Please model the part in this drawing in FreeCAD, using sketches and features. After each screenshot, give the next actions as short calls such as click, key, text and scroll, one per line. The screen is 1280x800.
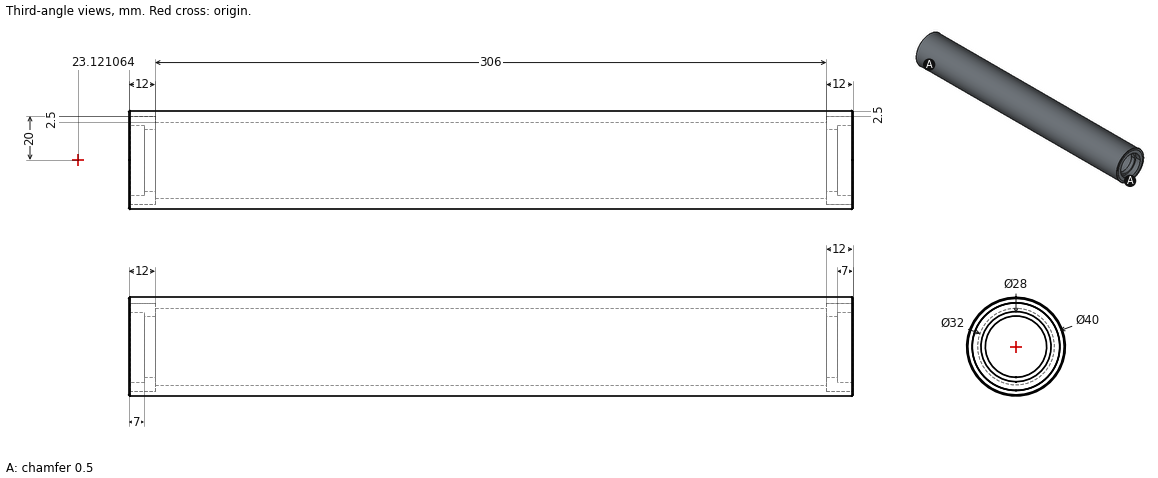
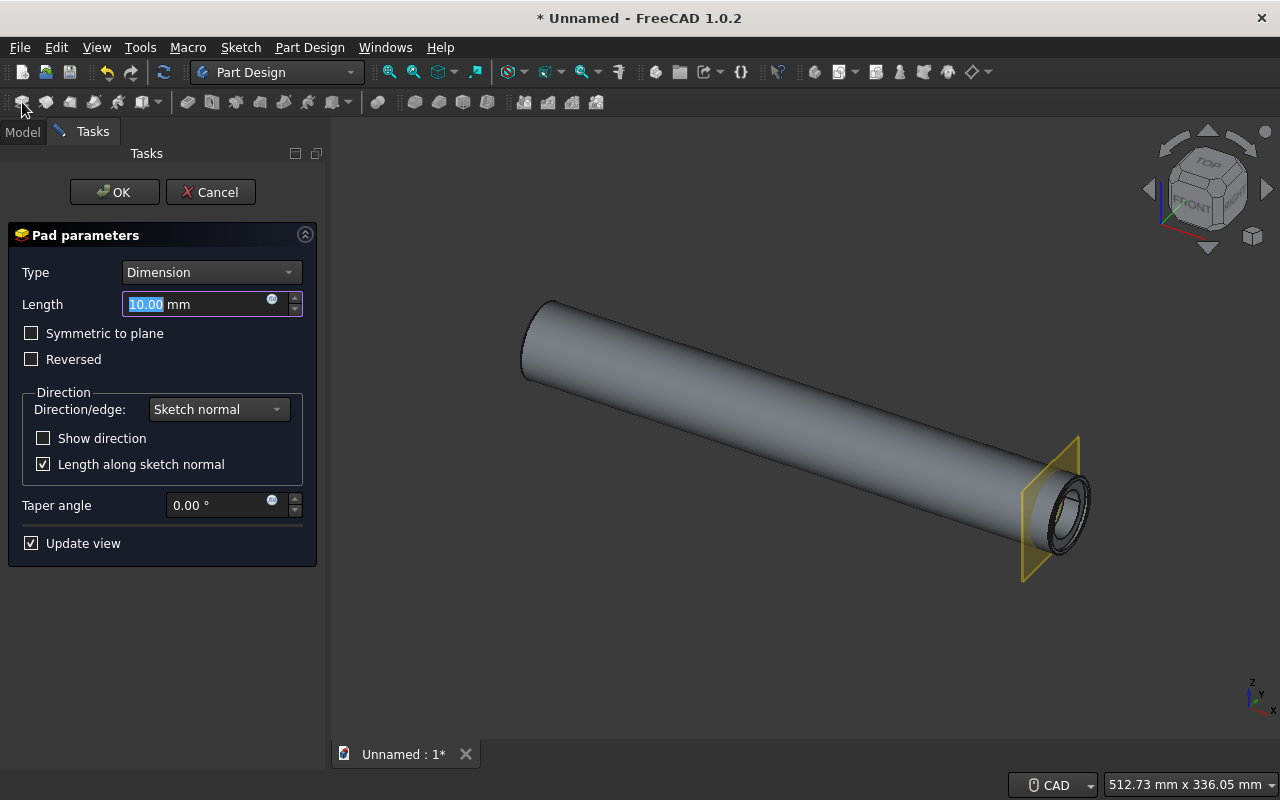
text(12)
key(Tab)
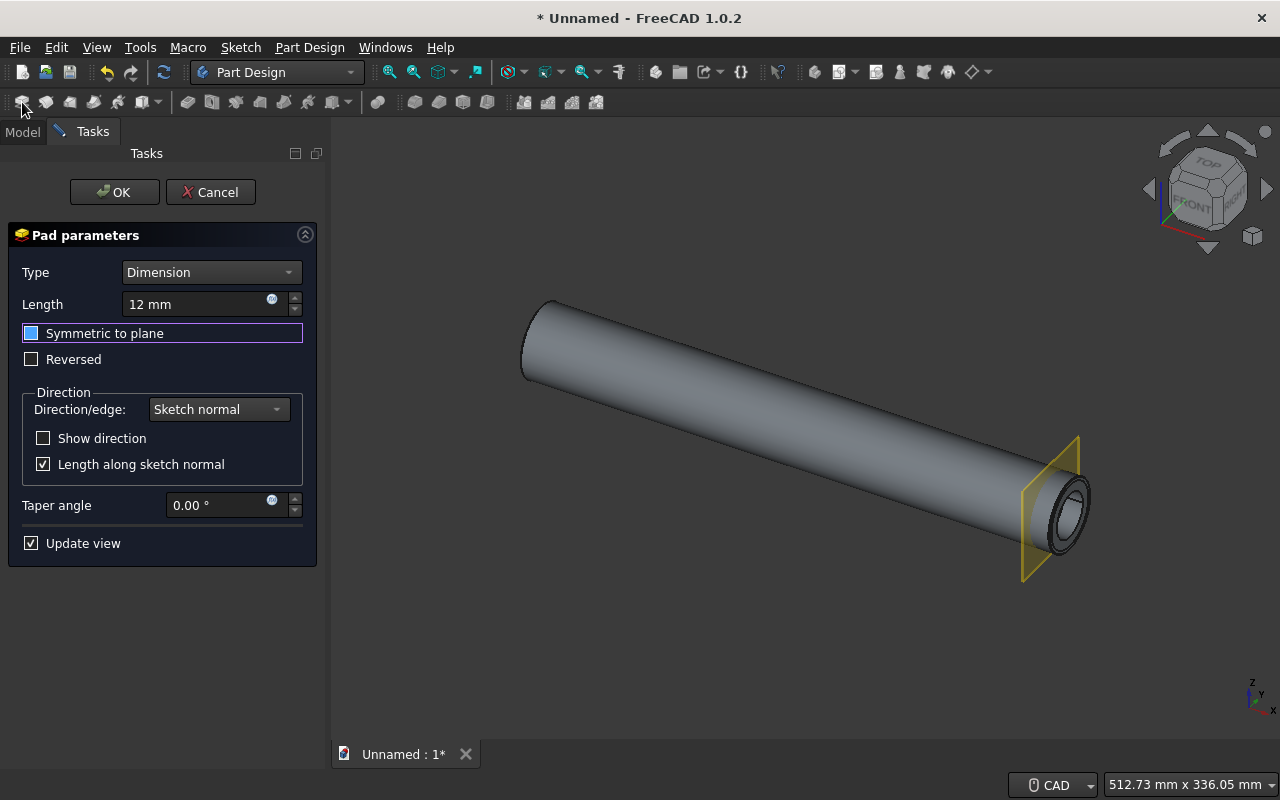
click(115, 192)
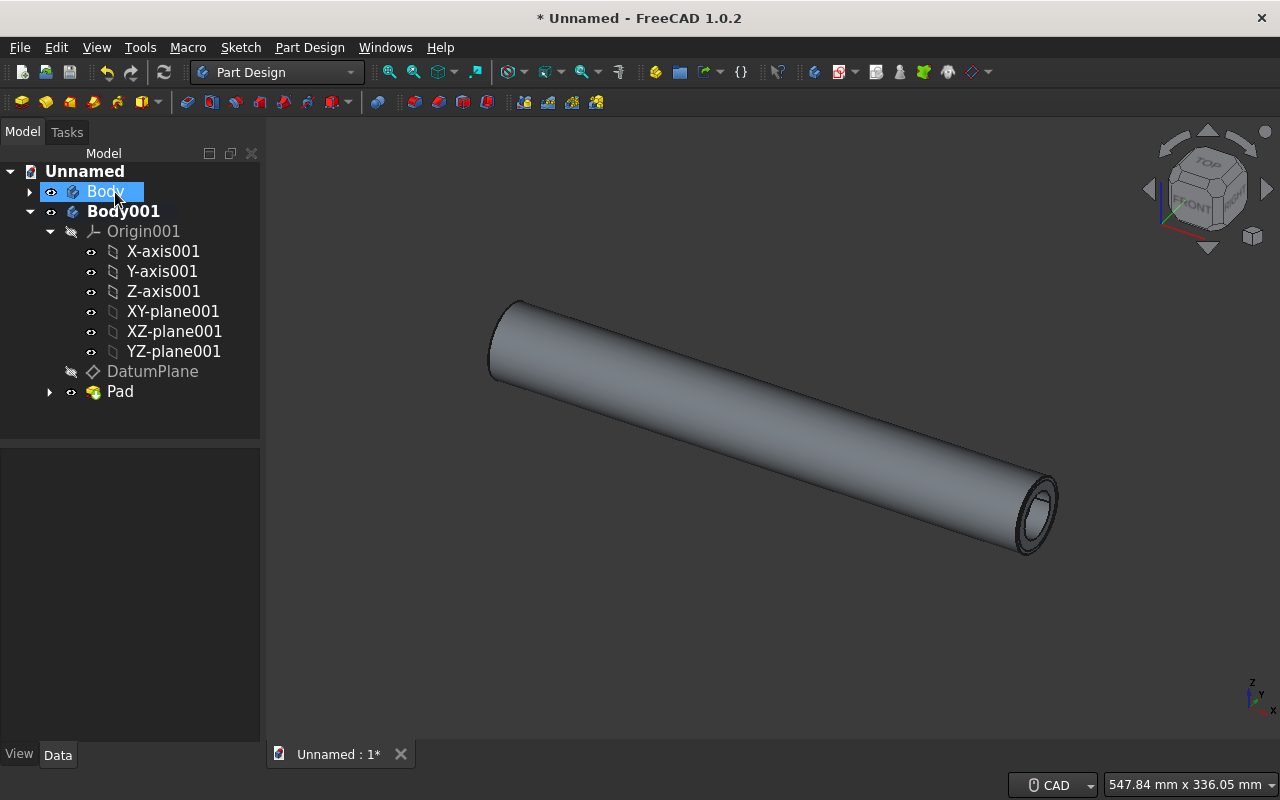
click(390, 72)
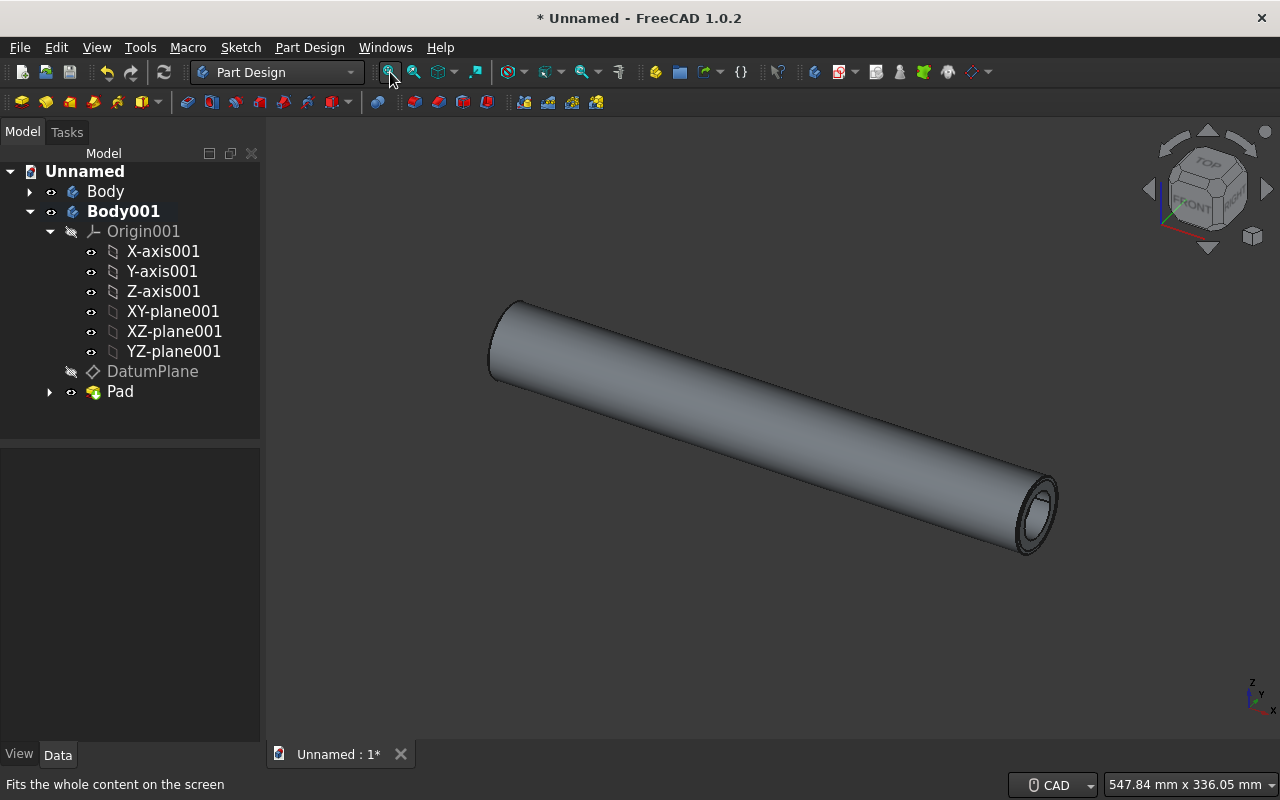
scroll(1037, 541, up, 5)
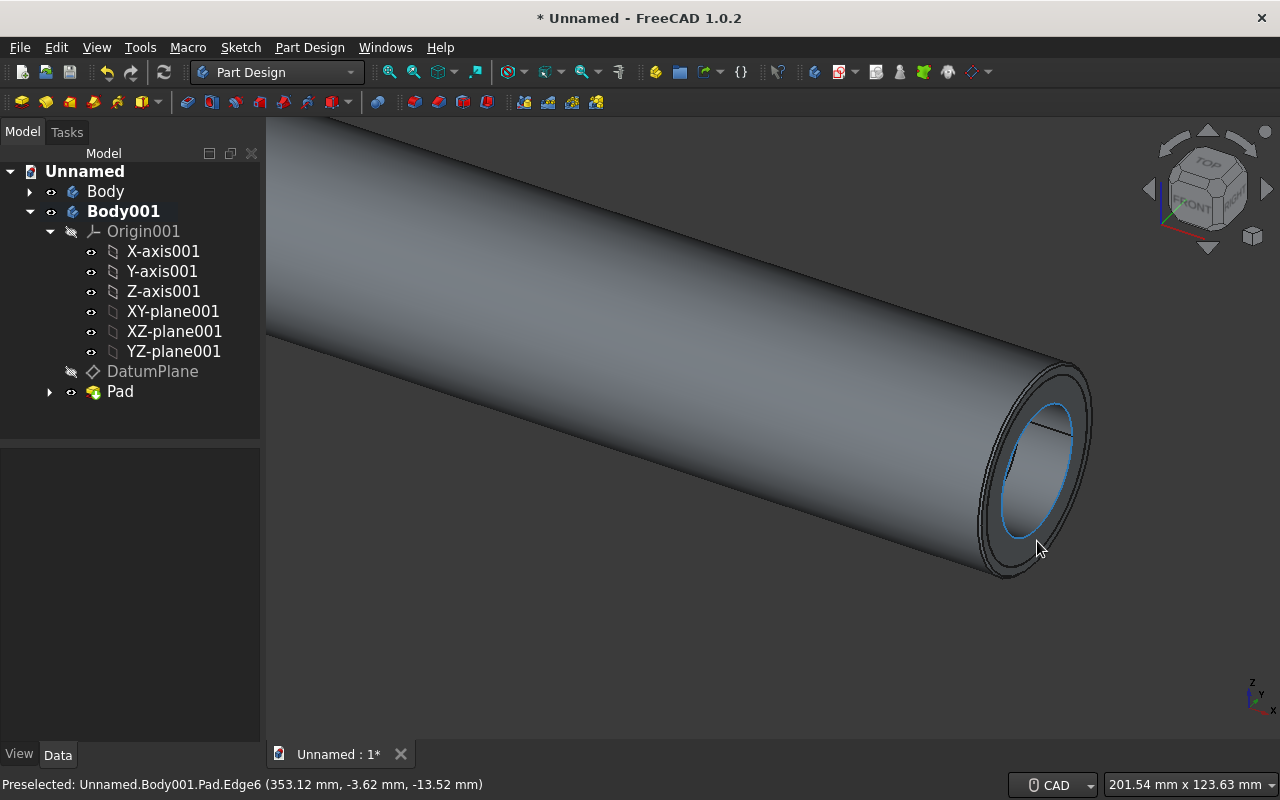
click(1037, 541)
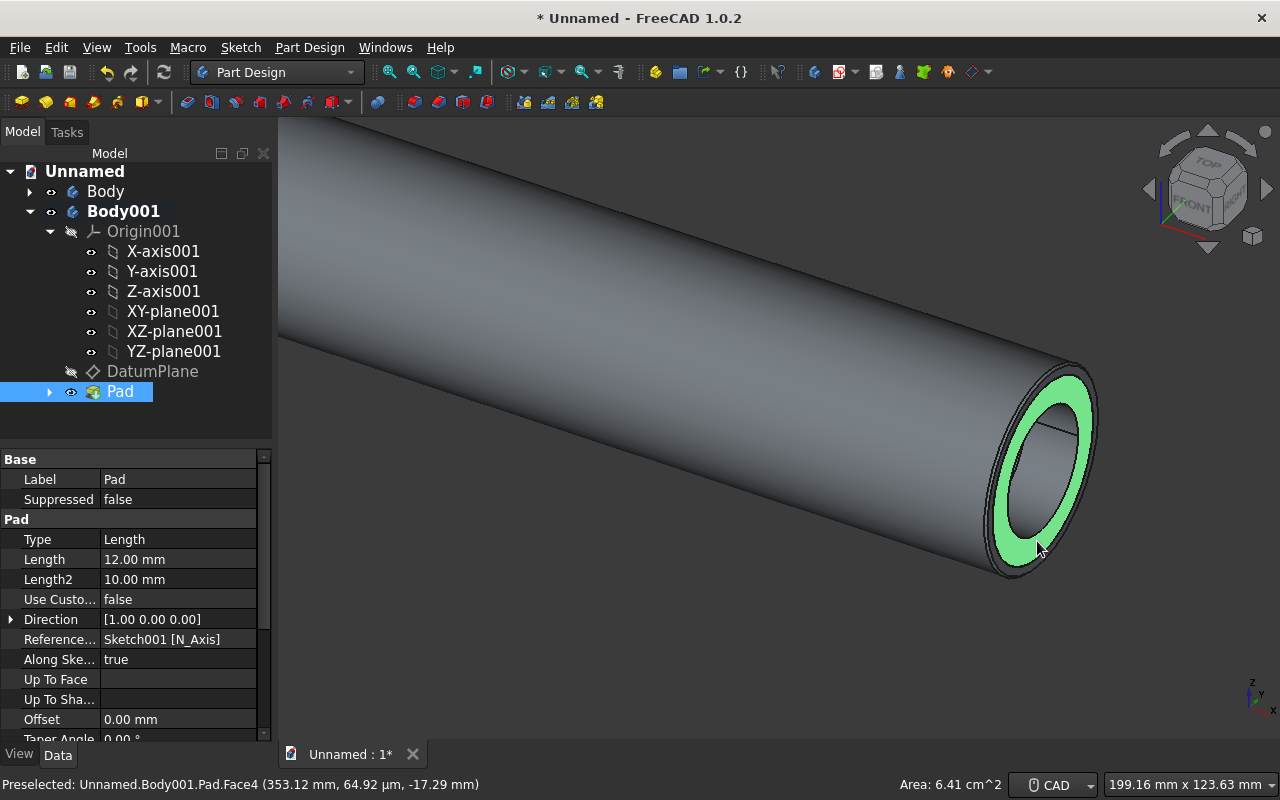
click(840, 72)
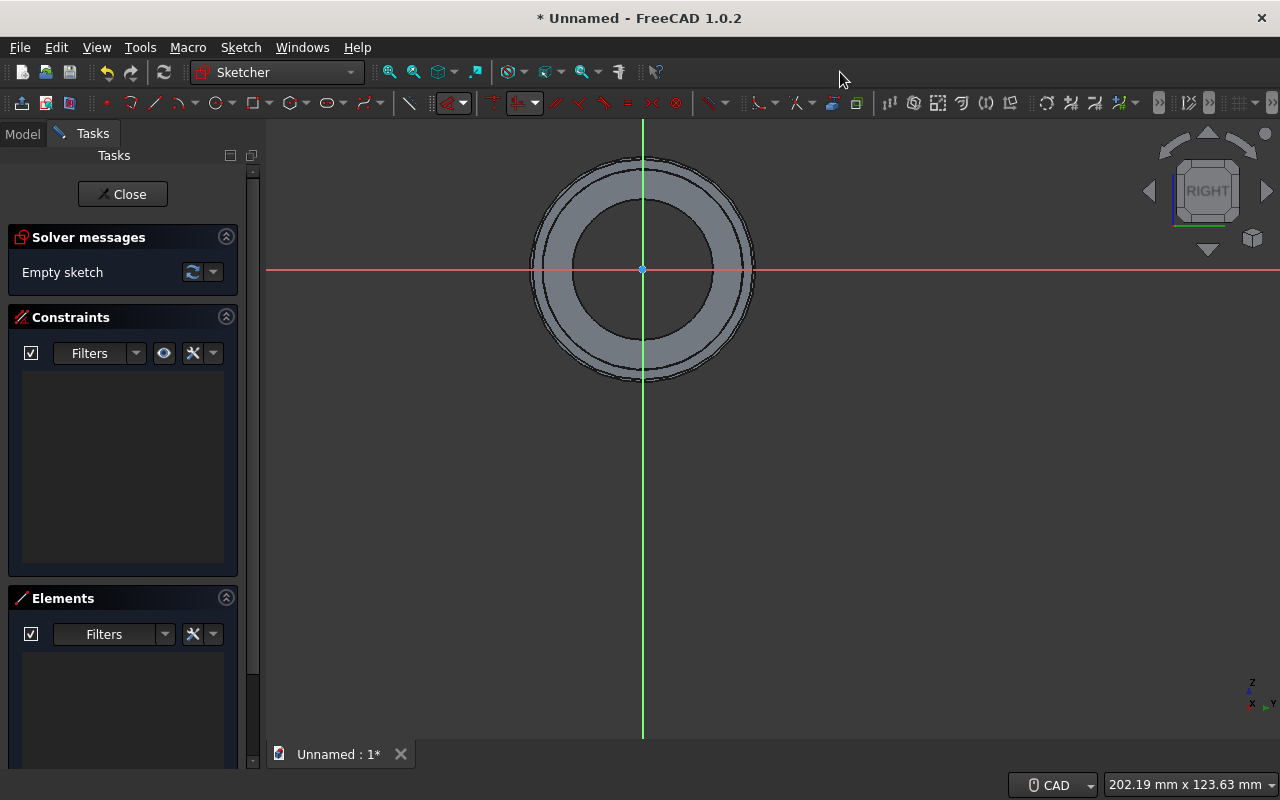
scroll(607, 177, up, 5)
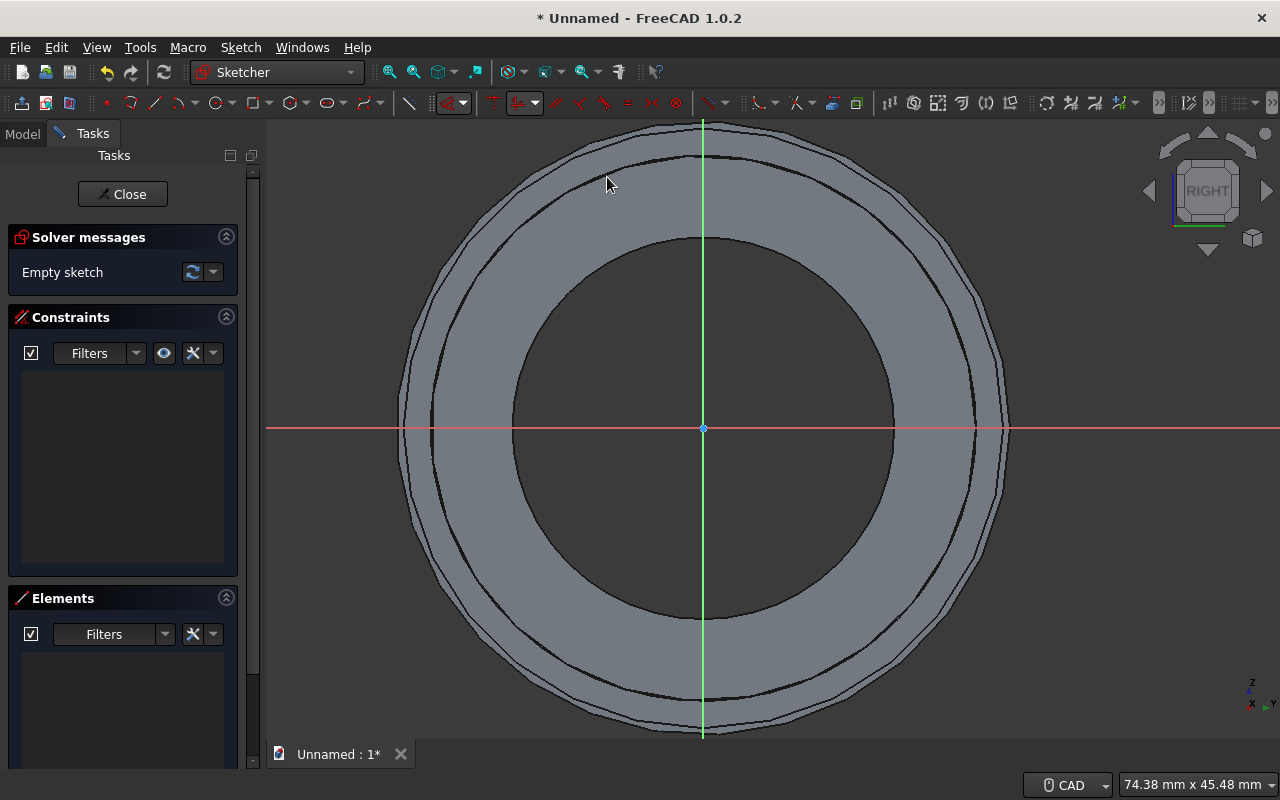
click(216, 104)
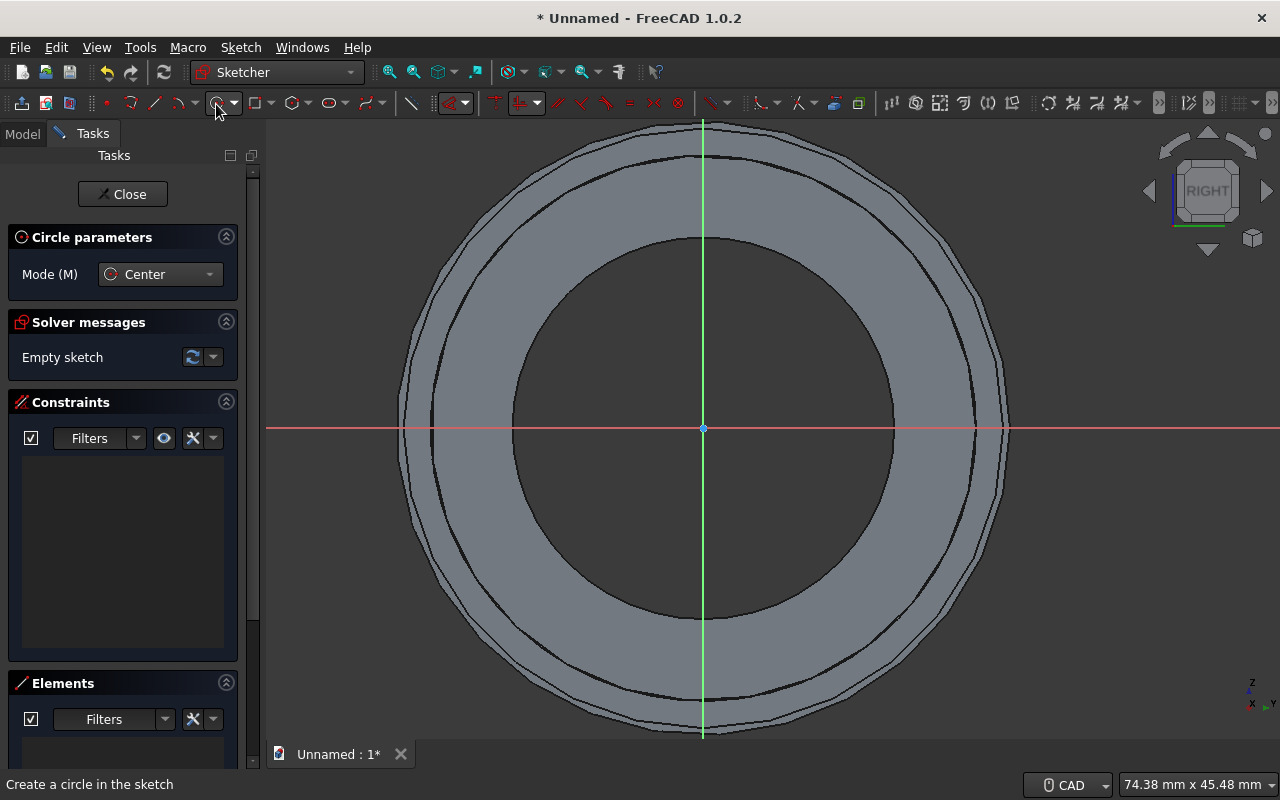
click(703, 428)
move(858, 274)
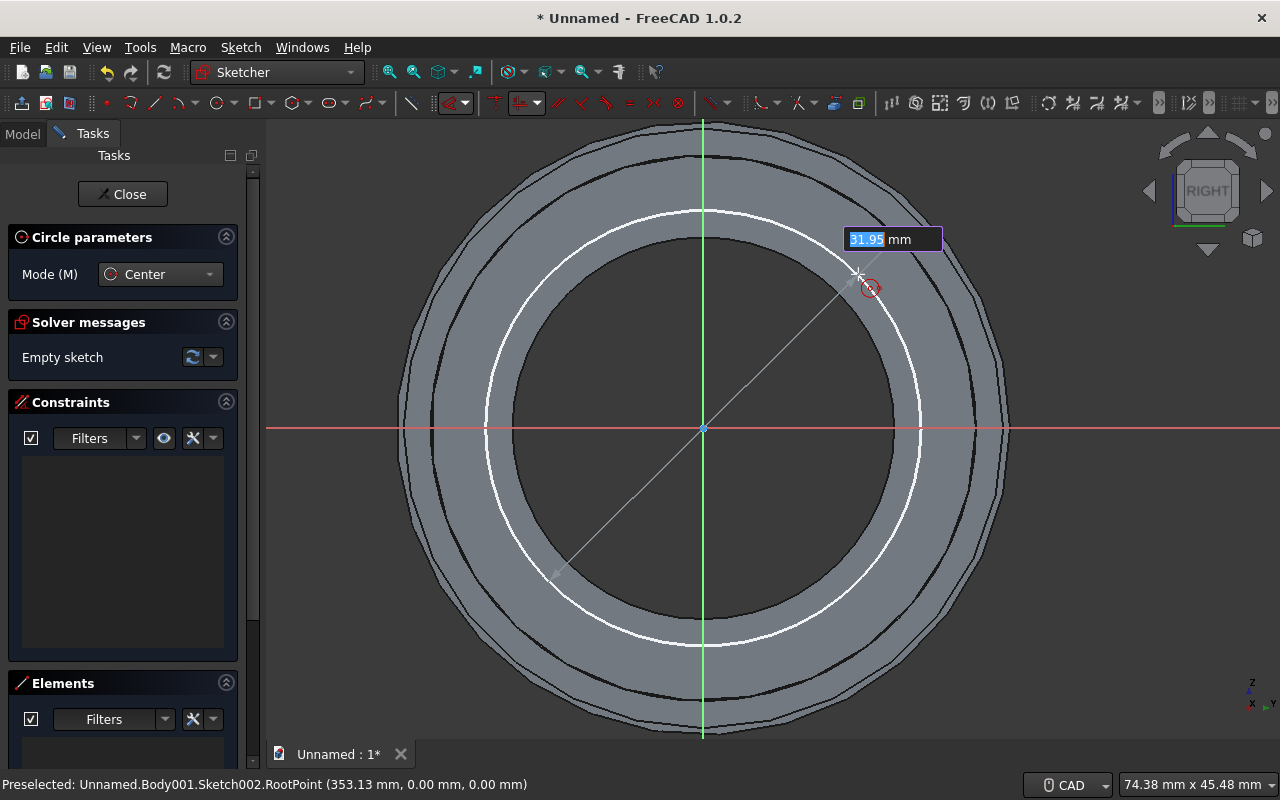
text(32)
key(Return)
key(Escape)